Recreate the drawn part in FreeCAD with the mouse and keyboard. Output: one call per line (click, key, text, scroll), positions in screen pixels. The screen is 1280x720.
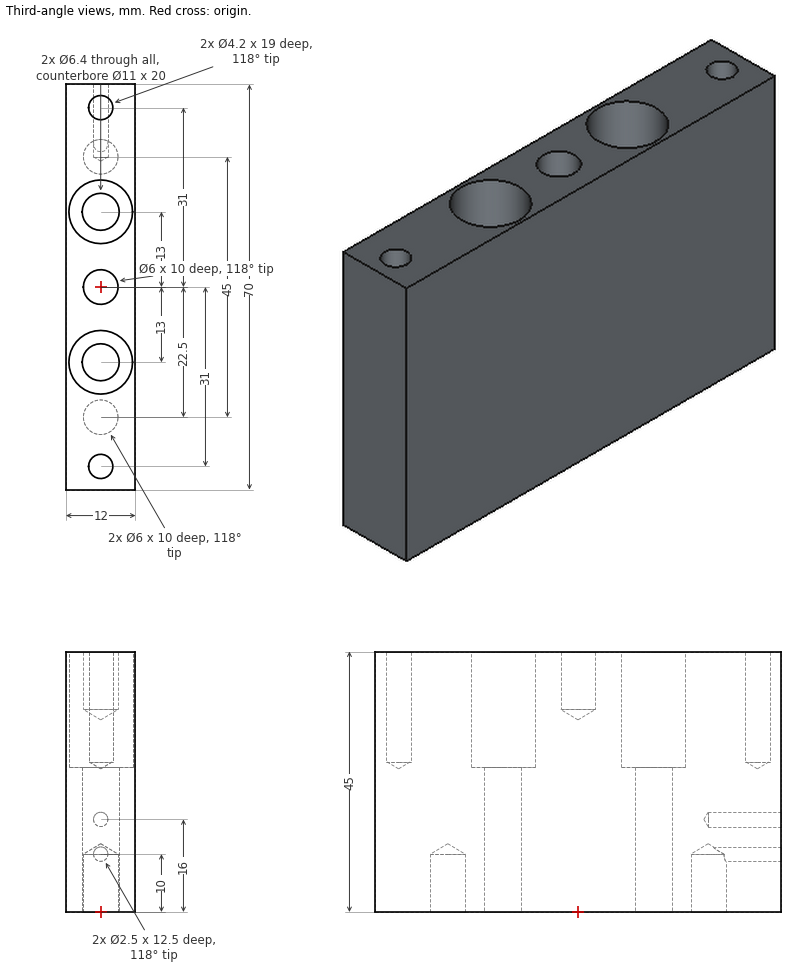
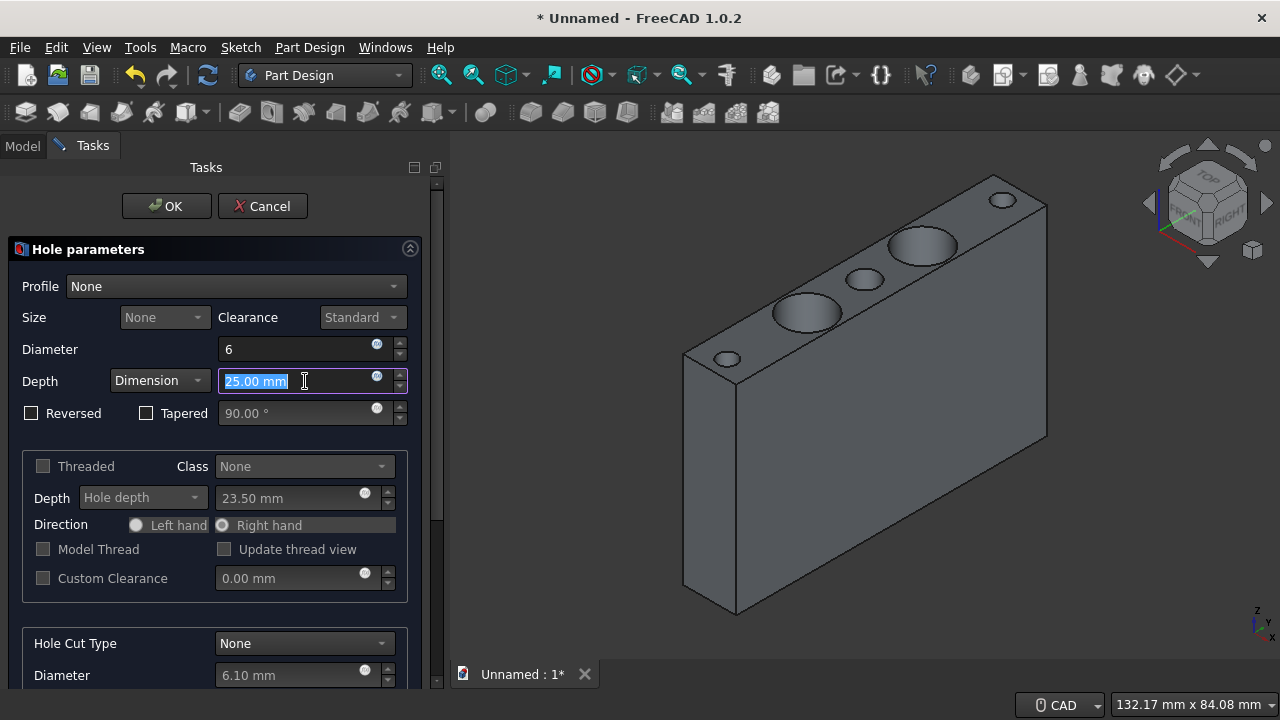
text(10)
key(Tab)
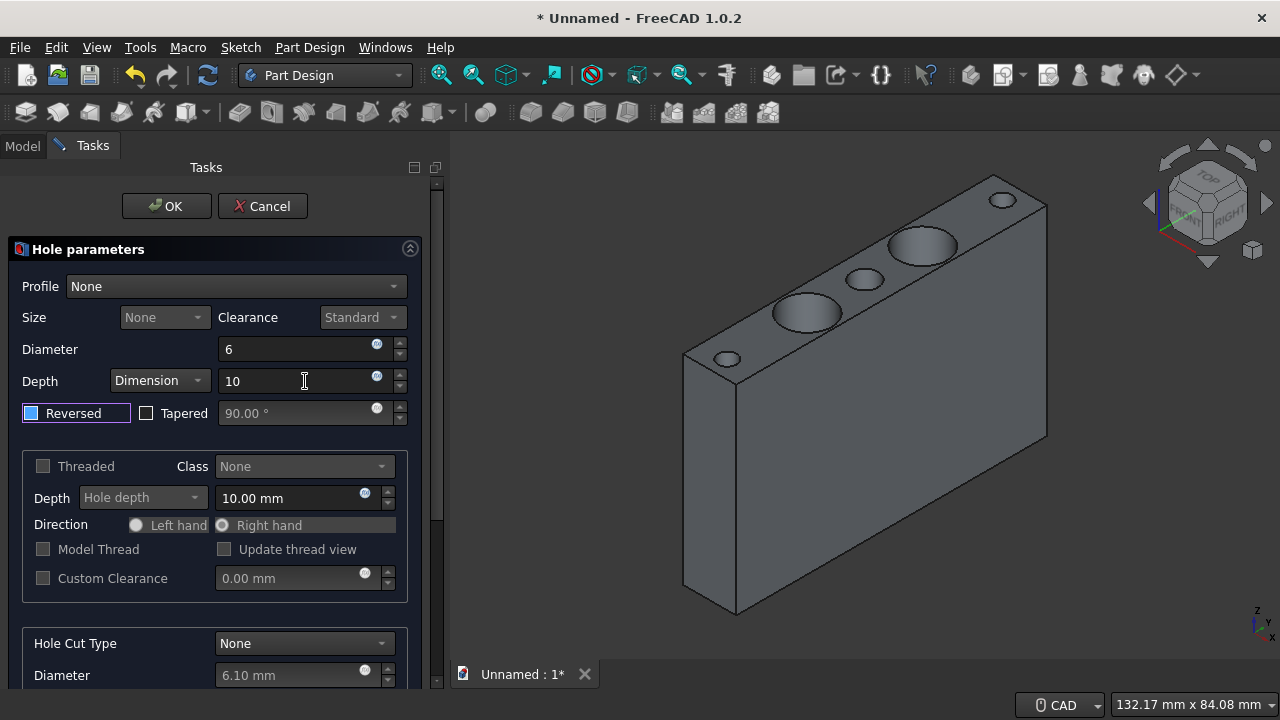
click(30, 413)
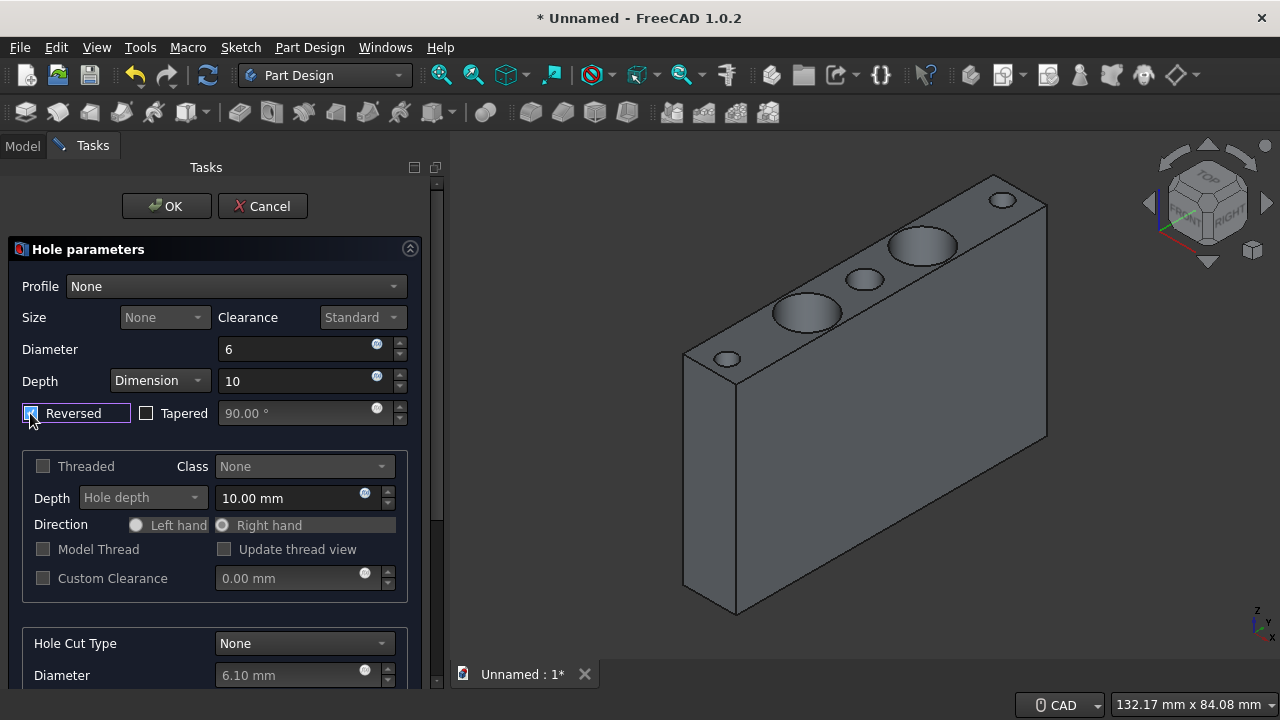
click(167, 206)